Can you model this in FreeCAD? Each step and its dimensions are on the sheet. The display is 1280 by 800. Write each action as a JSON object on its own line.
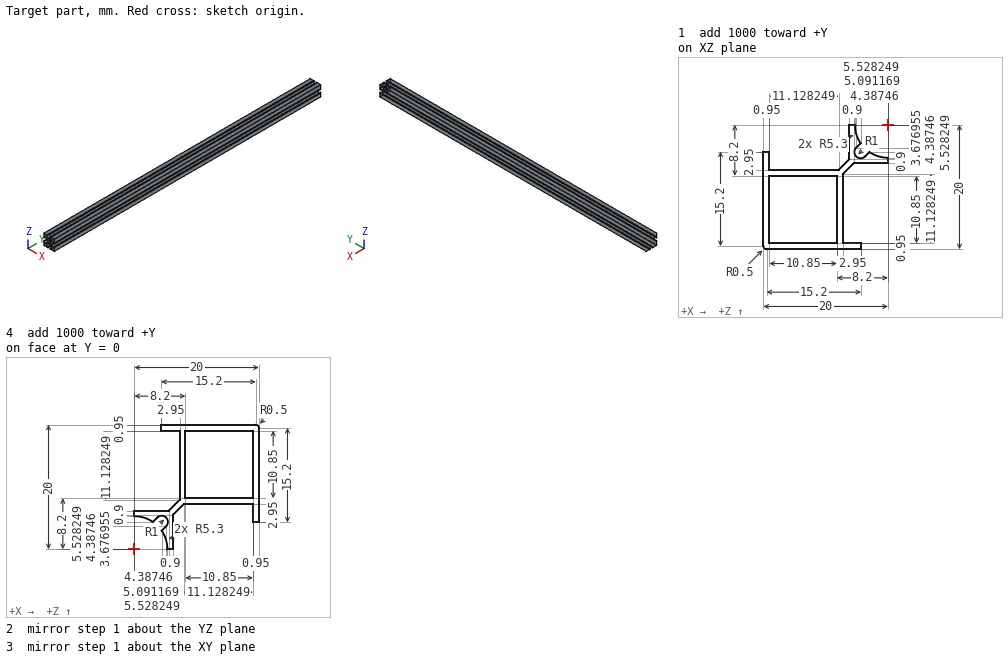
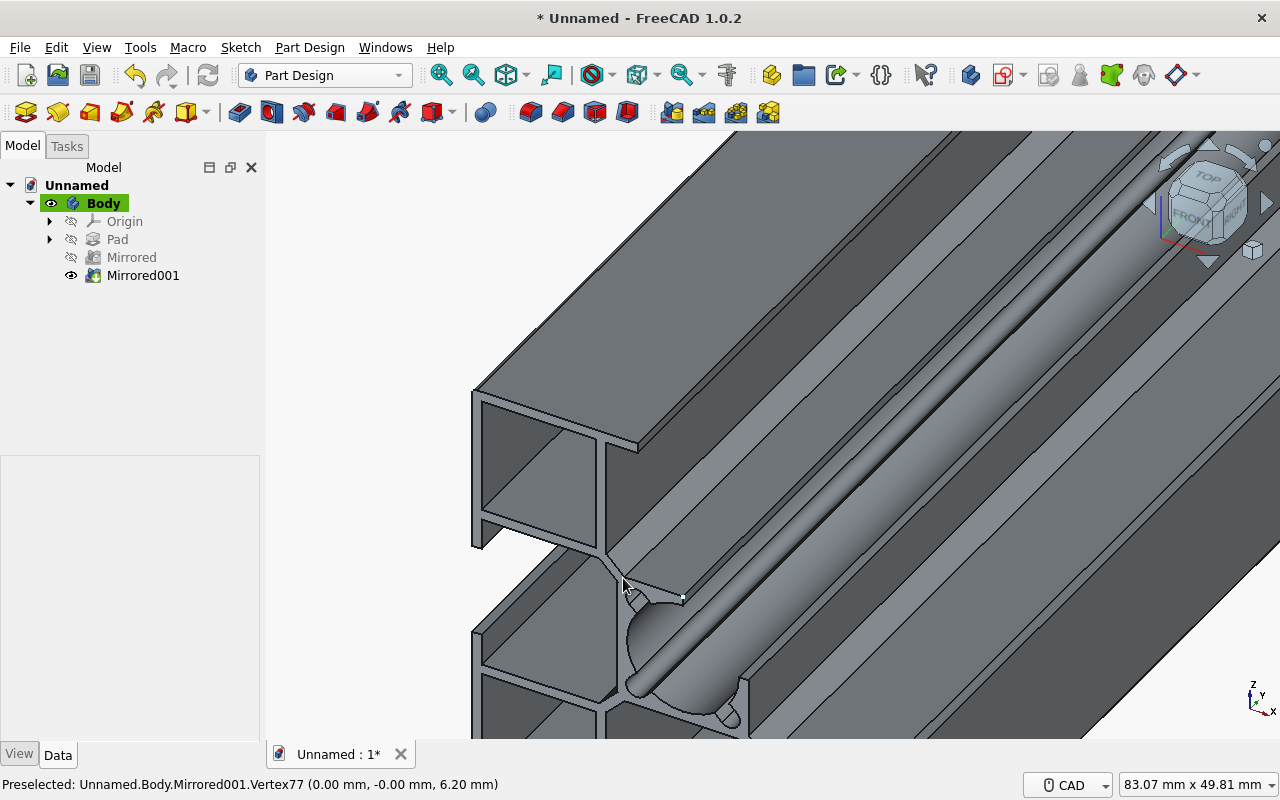
{"action": "scroll", "coordinate": [623, 580], "scroll_direction": "up", "scroll_amount": 4}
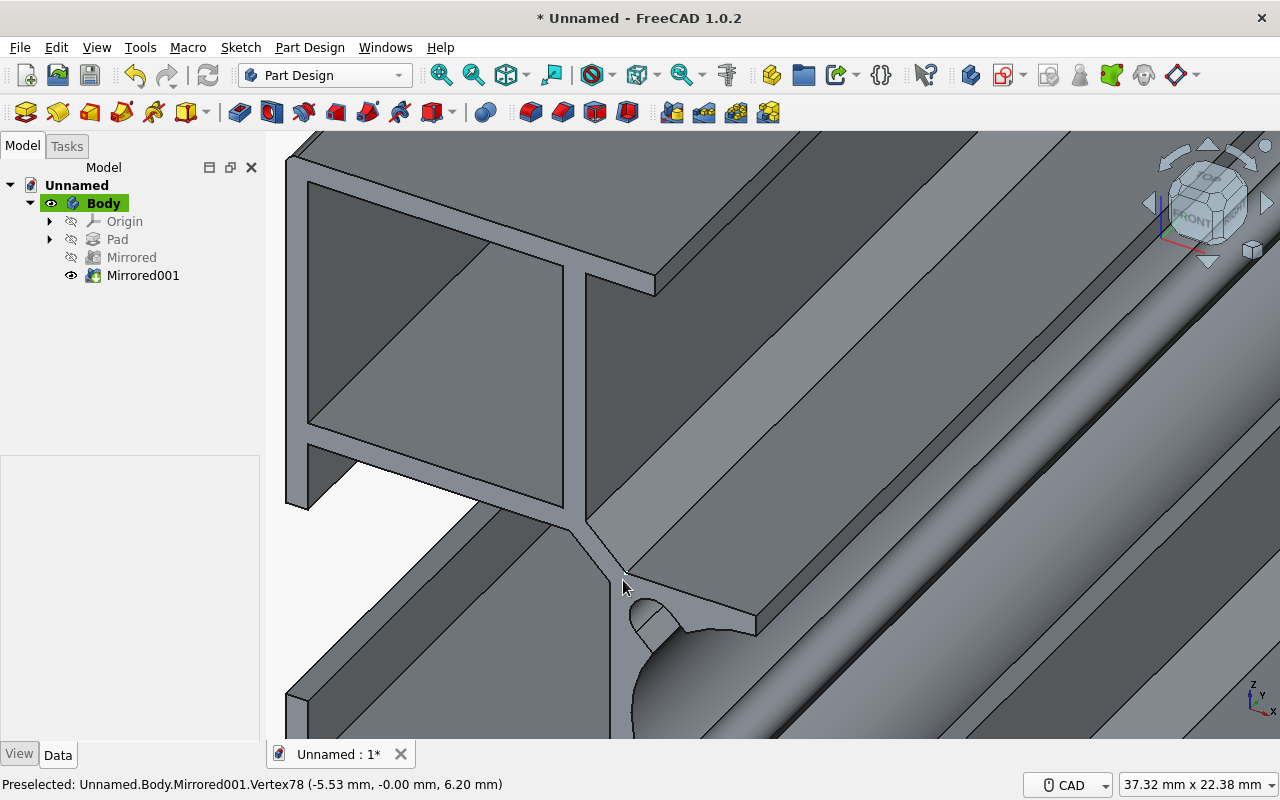
{"action": "left_click", "coordinate": [622, 581]}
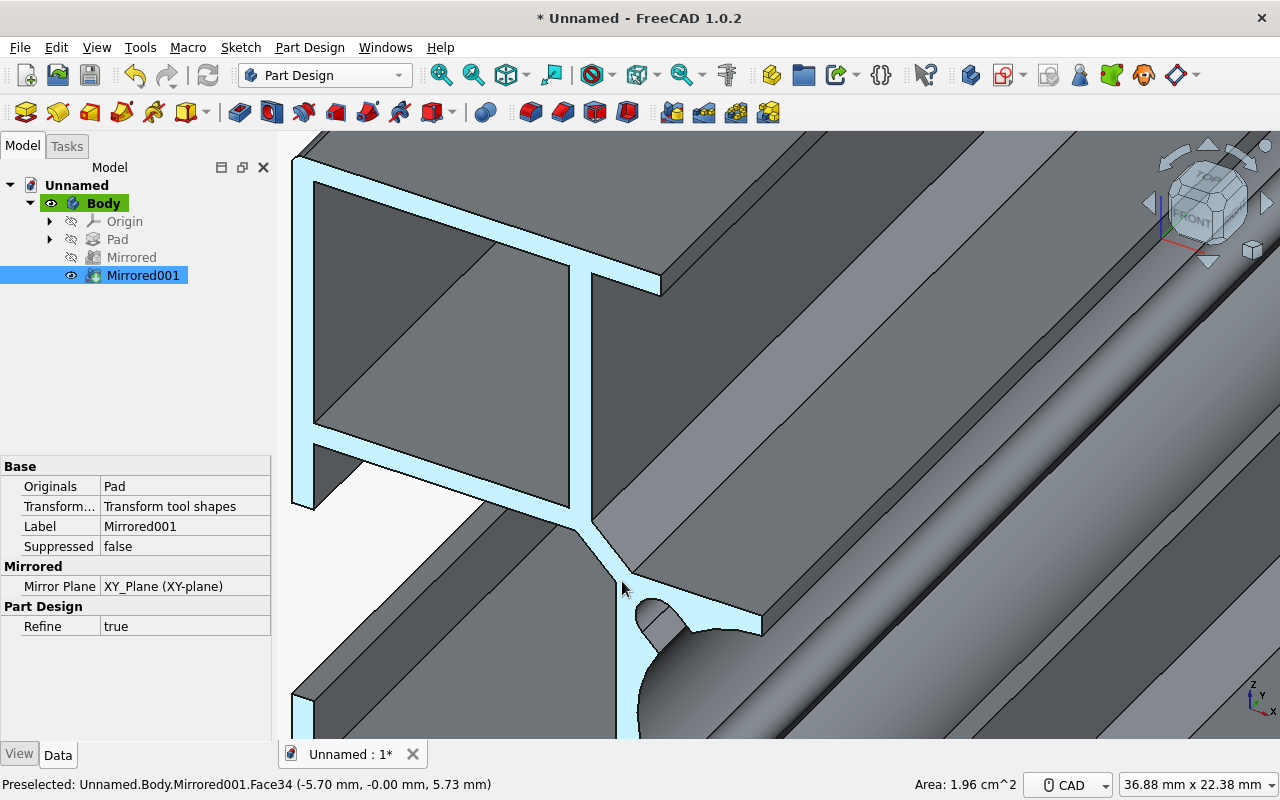
{"action": "left_click", "coordinate": [1004, 76]}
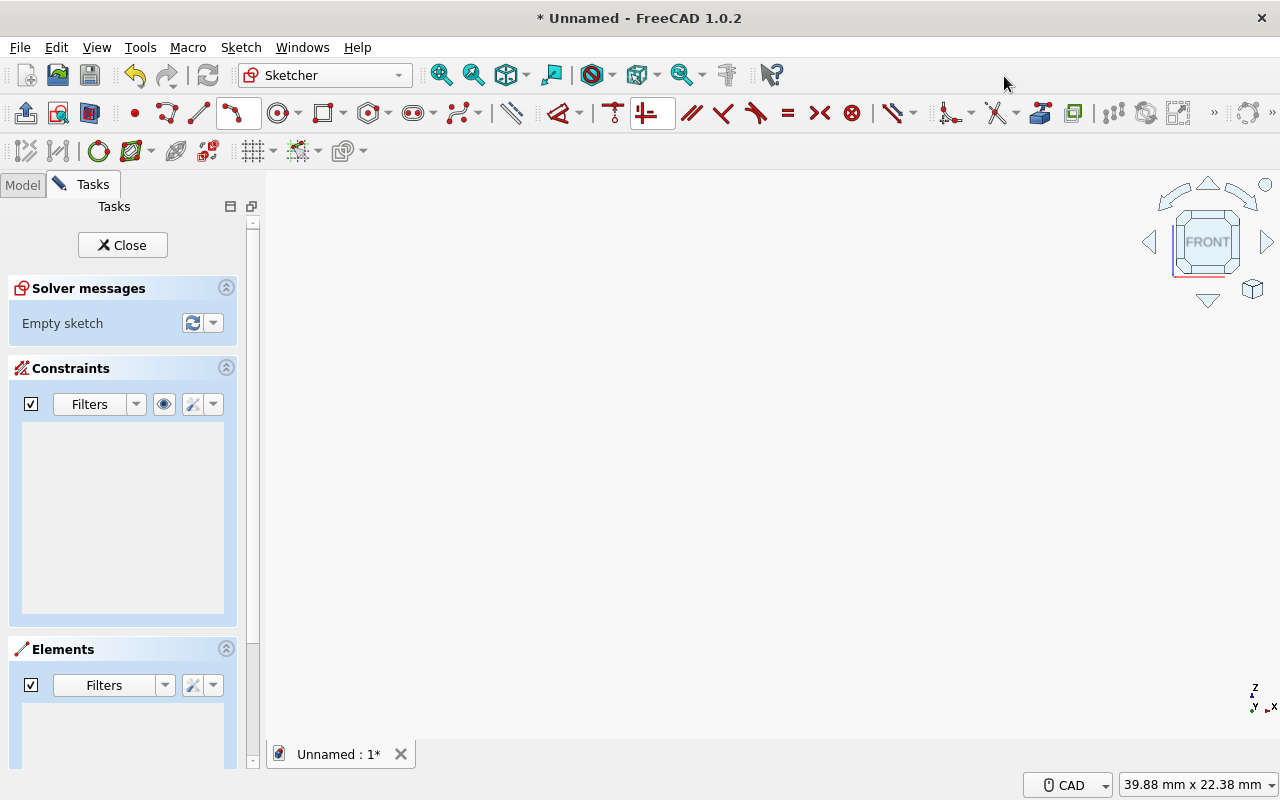
{"action": "scroll", "coordinate": [704, 454], "scroll_direction": "down", "scroll_amount": 5}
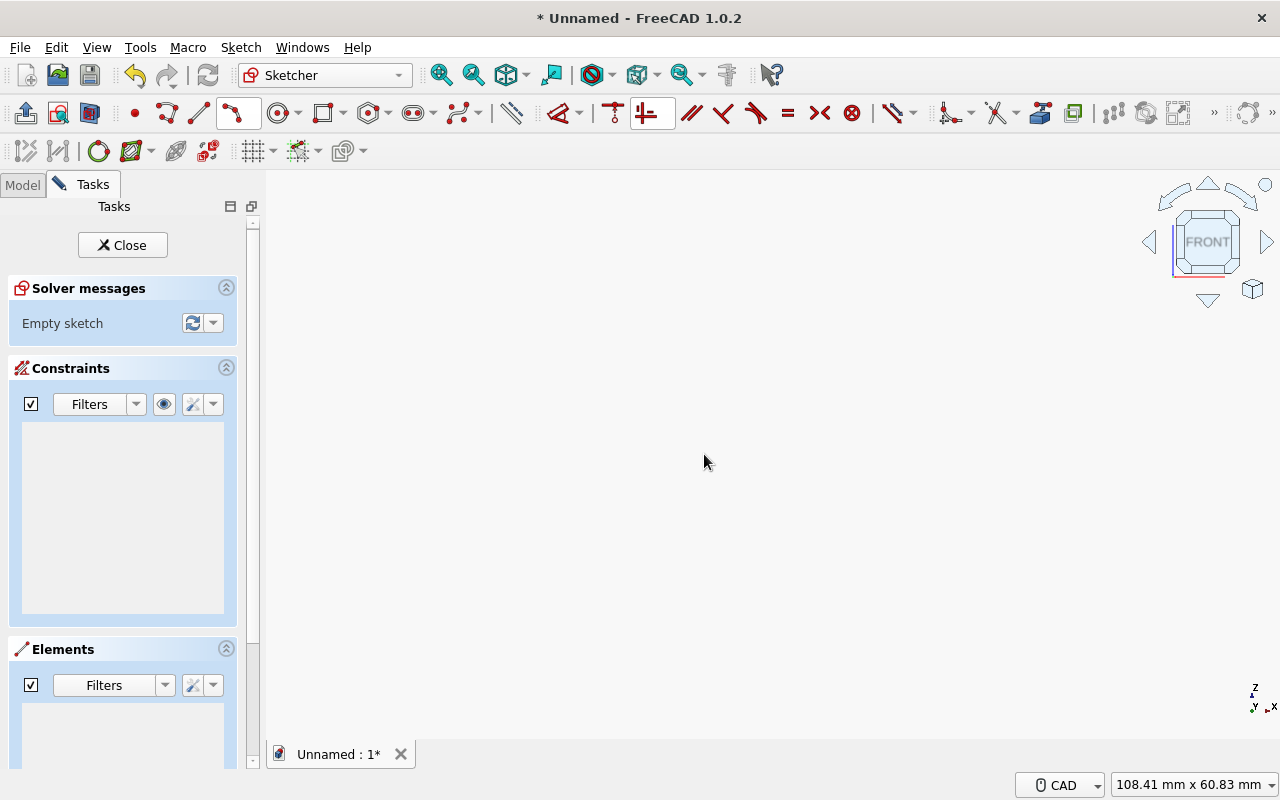
{"action": "scroll", "coordinate": [704, 454], "scroll_direction": "down", "scroll_amount": 5}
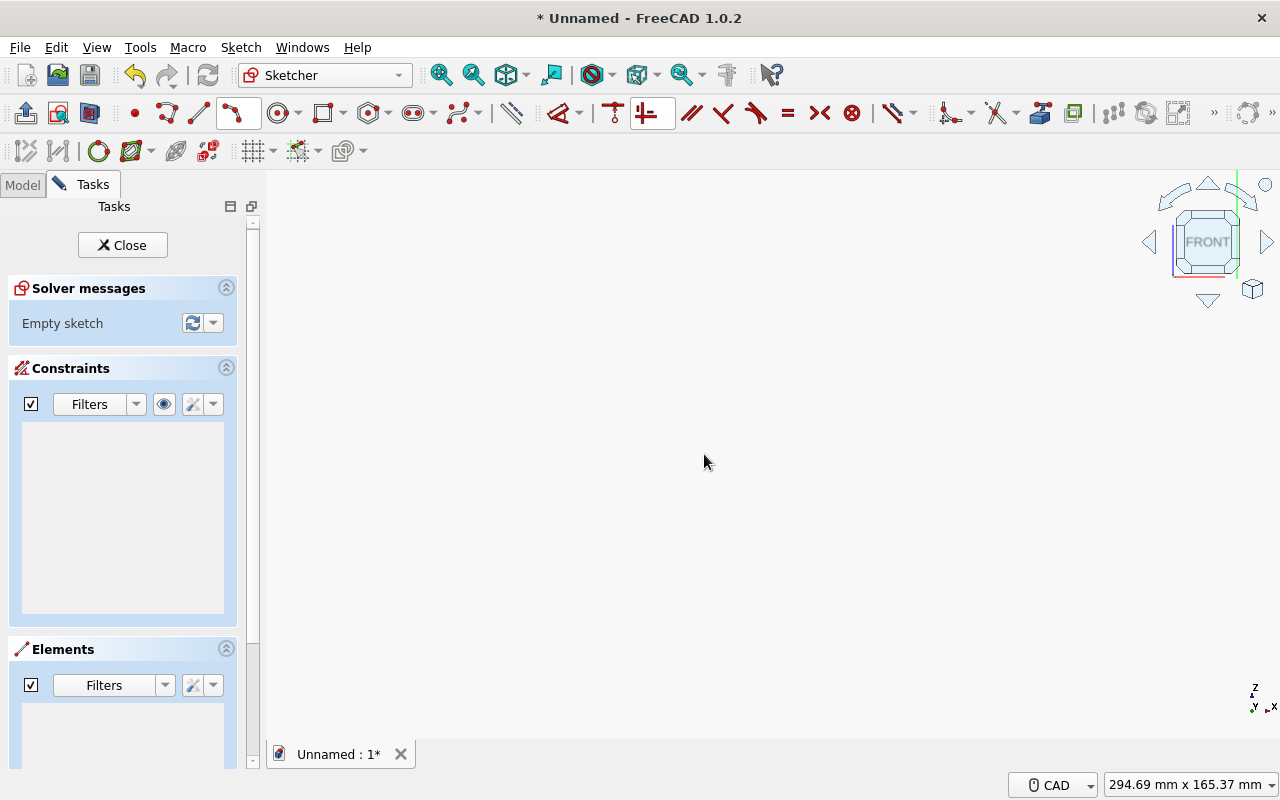
{"action": "scroll", "coordinate": [704, 454], "scroll_direction": "down", "scroll_amount": 5}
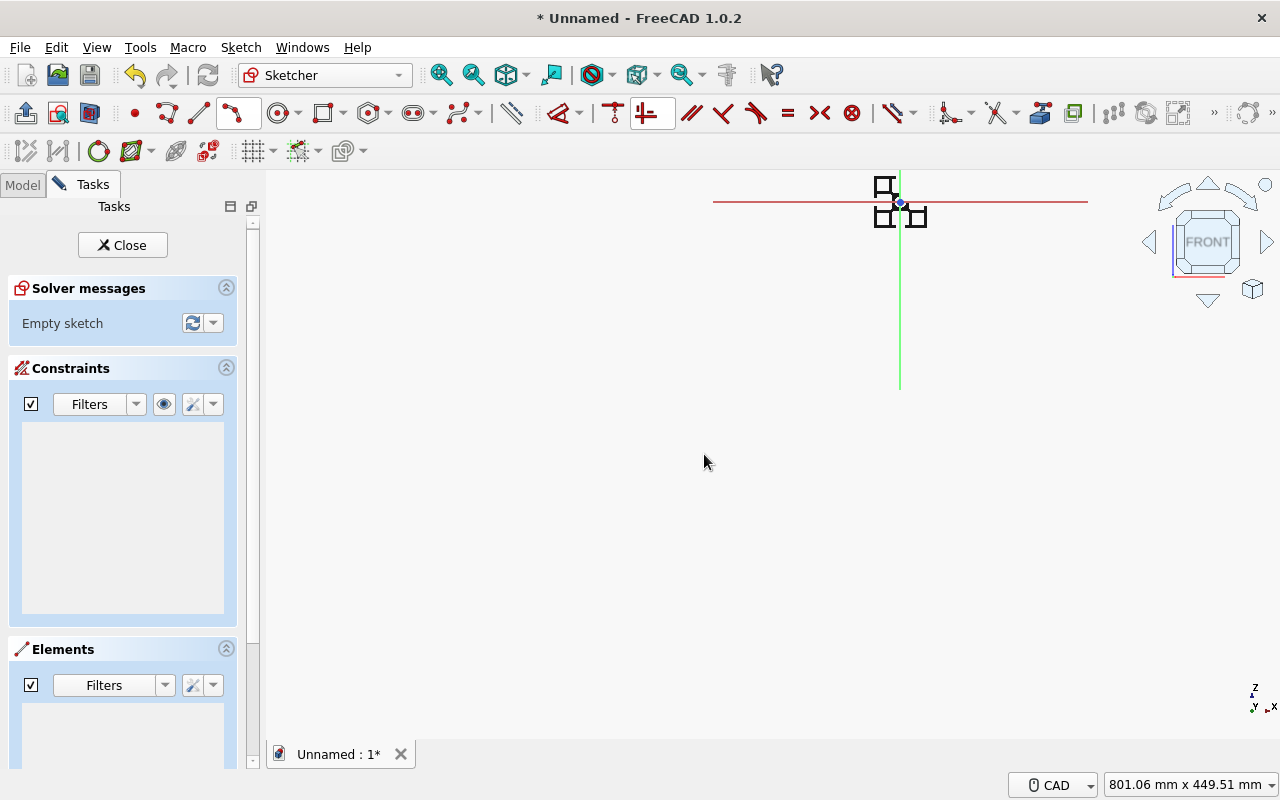
{"action": "scroll", "coordinate": [704, 454], "scroll_direction": "down", "scroll_amount": 5}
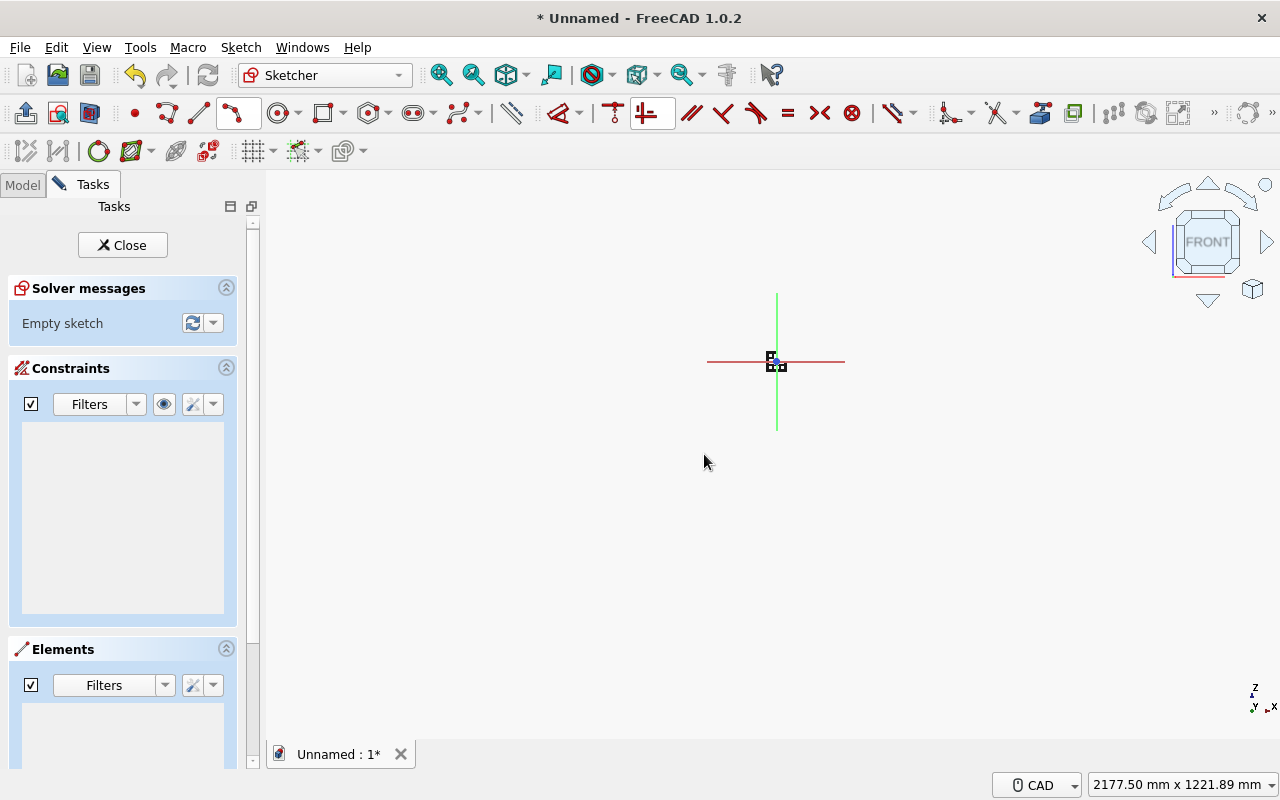
{"action": "scroll", "coordinate": [785, 352], "scroll_direction": "up", "scroll_amount": 15}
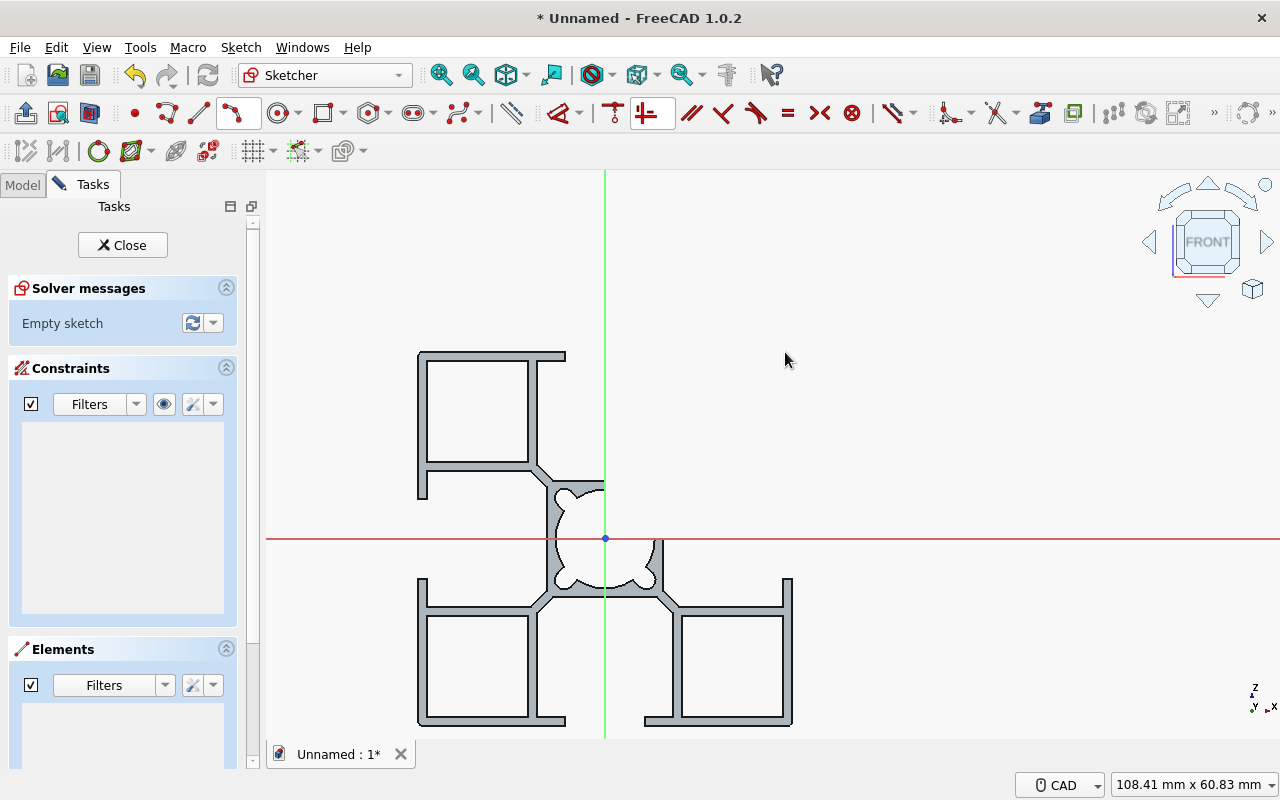
{"action": "key", "text": "g m"}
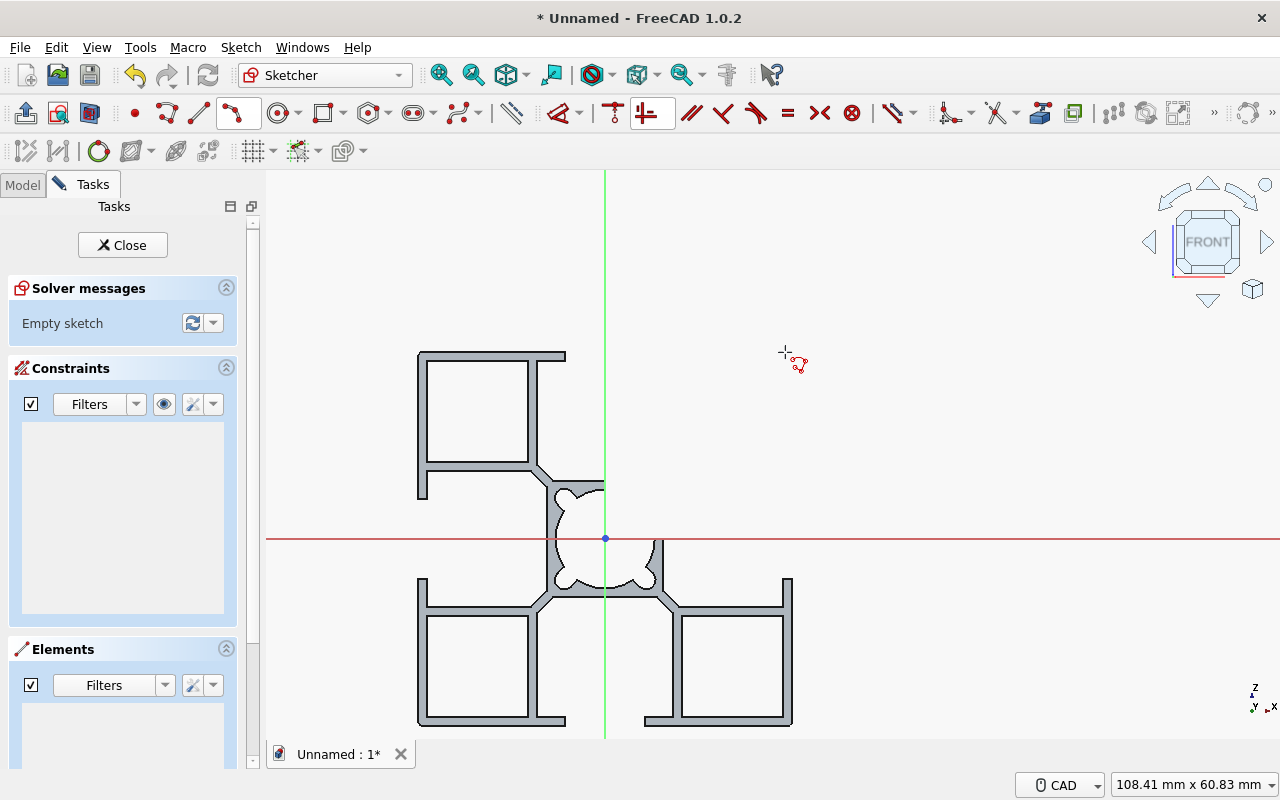
{"action": "left_click", "coordinate": [792, 357]}
{"action": "left_click", "coordinate": [792, 499]}